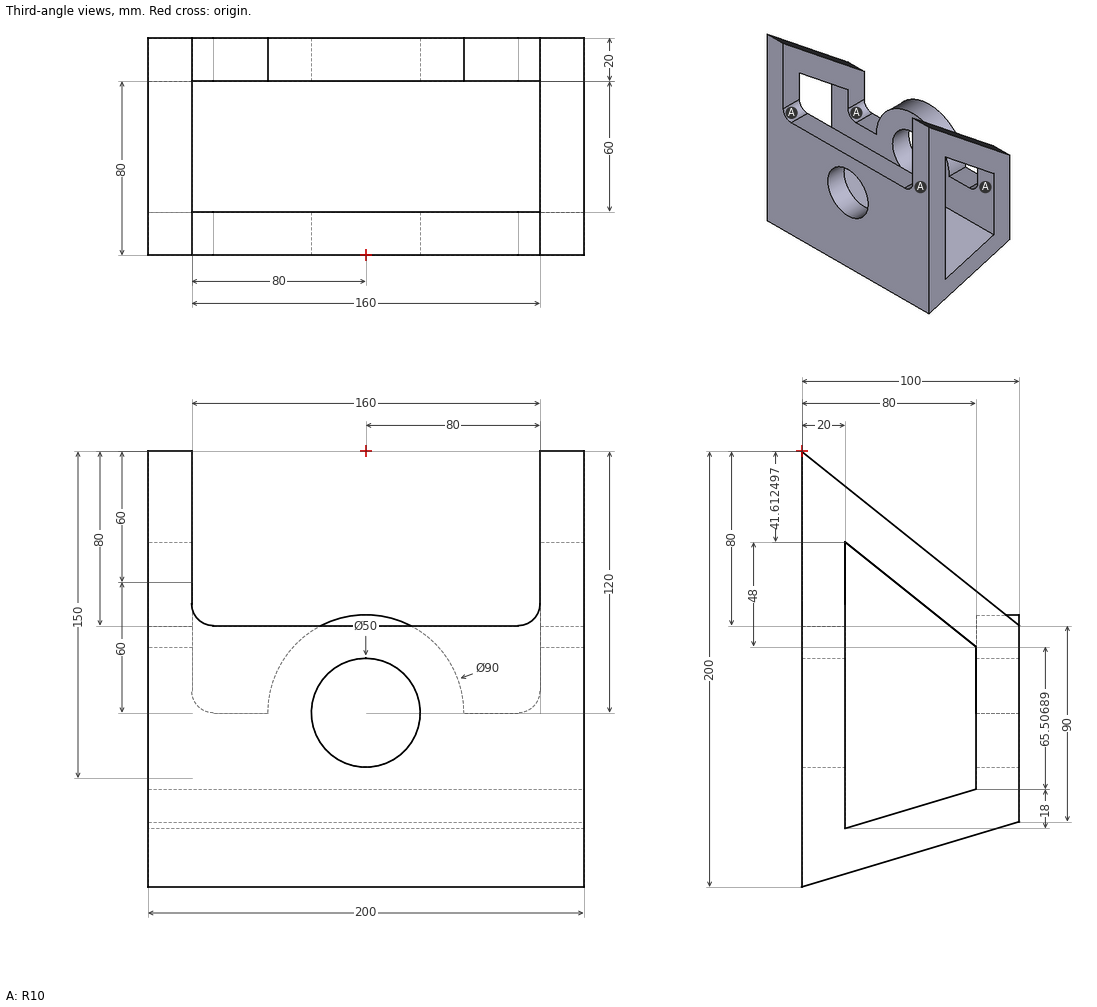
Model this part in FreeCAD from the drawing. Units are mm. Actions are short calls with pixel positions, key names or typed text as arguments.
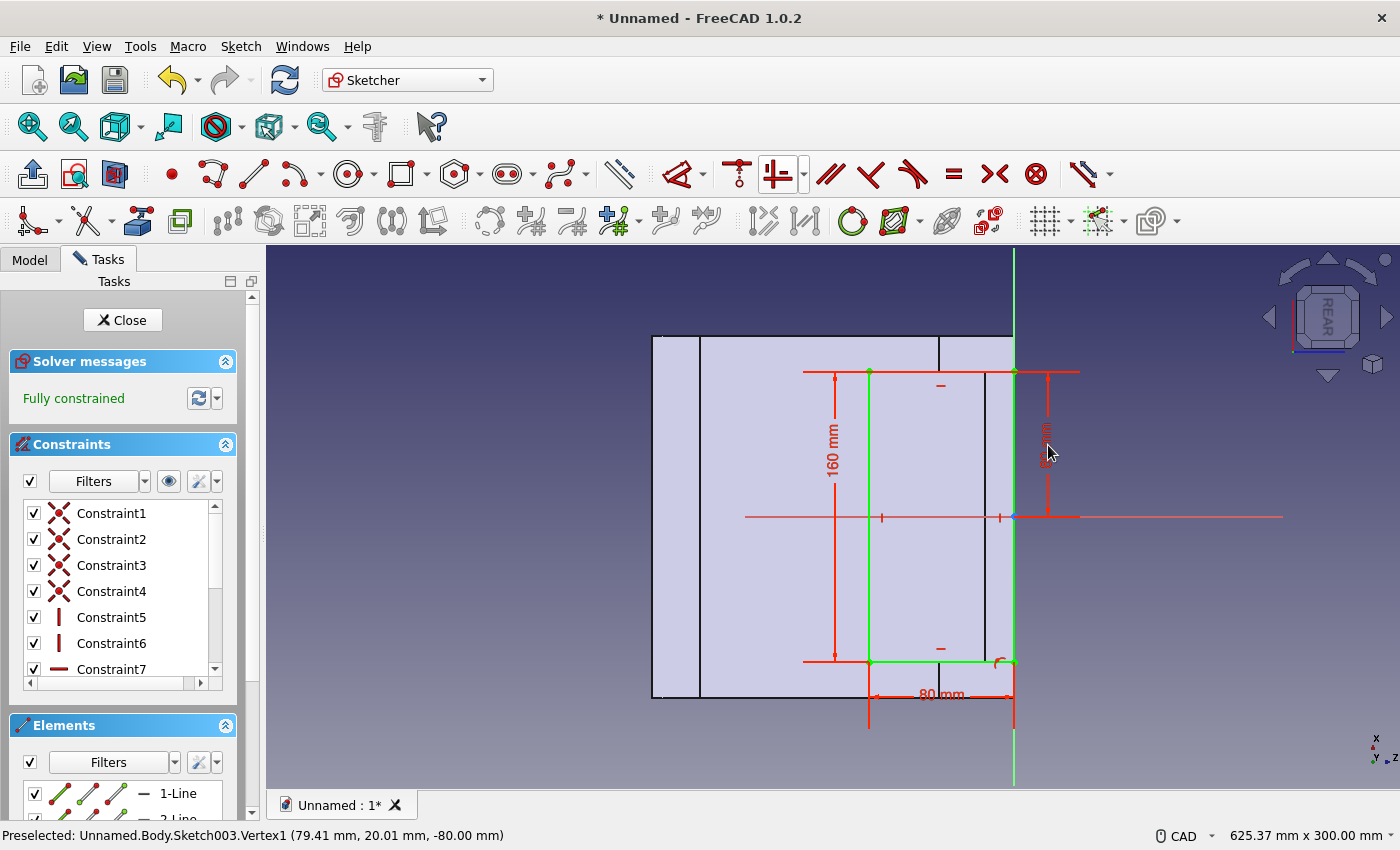
click(123, 320)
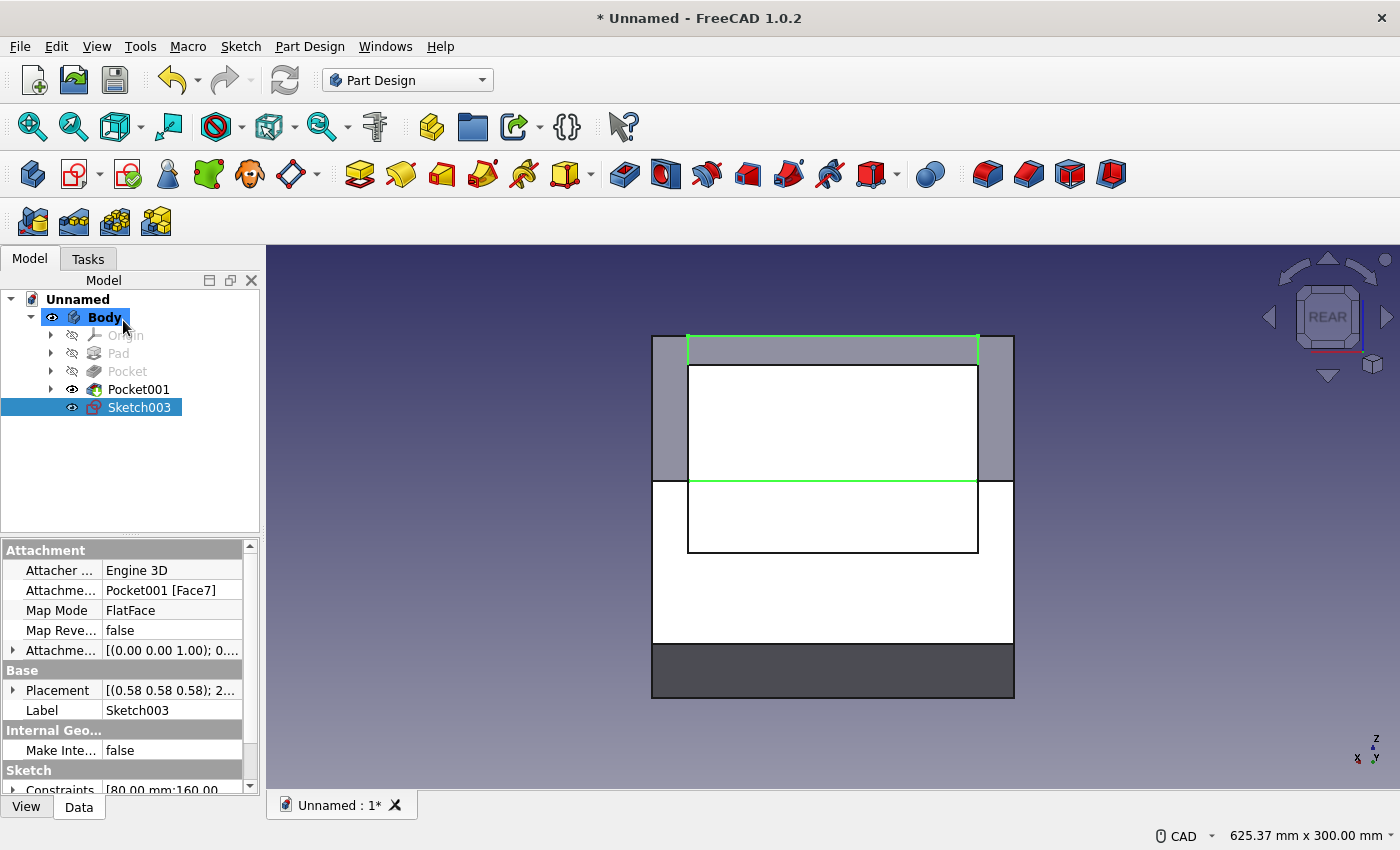
click(625, 174)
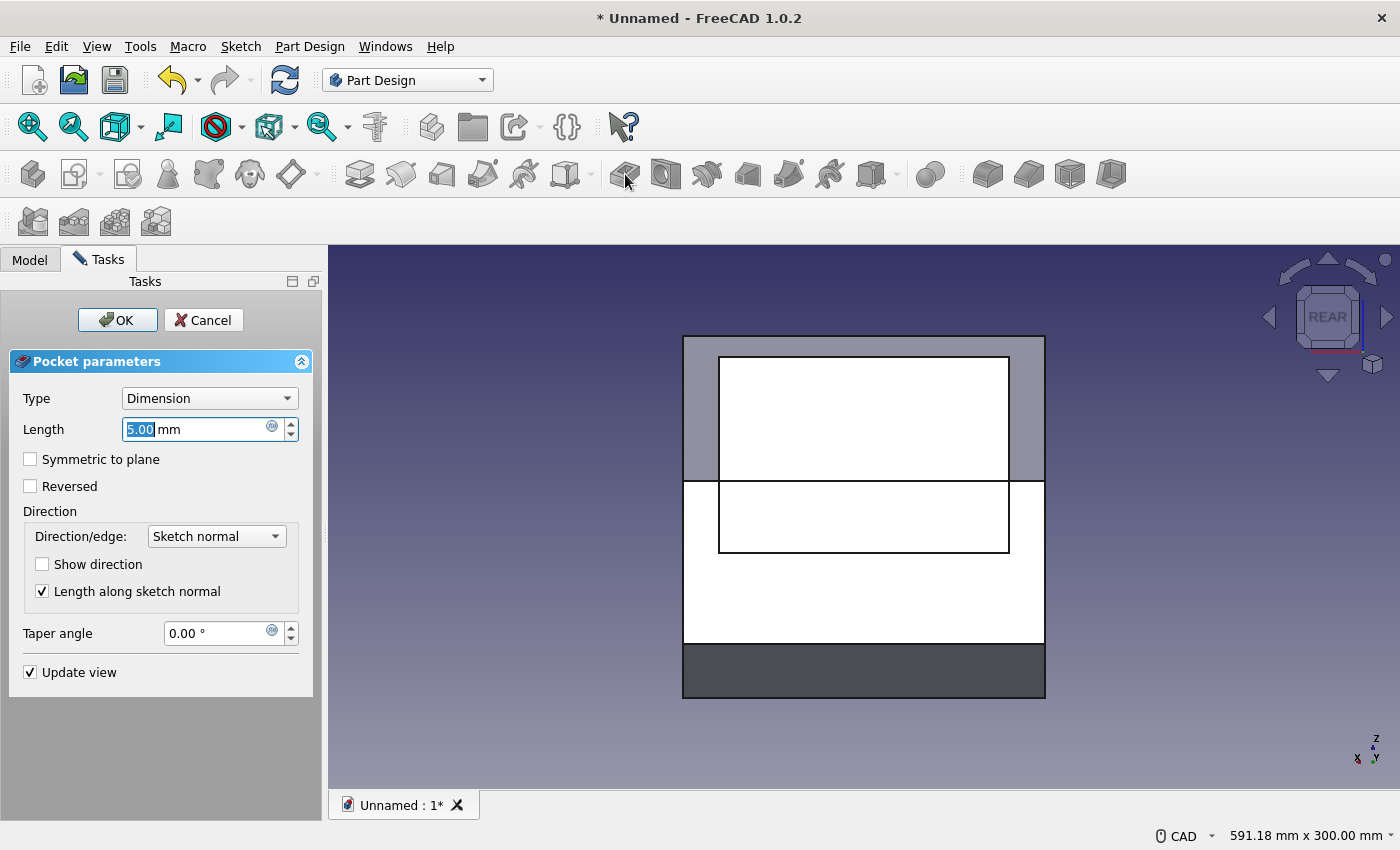
click(210, 398)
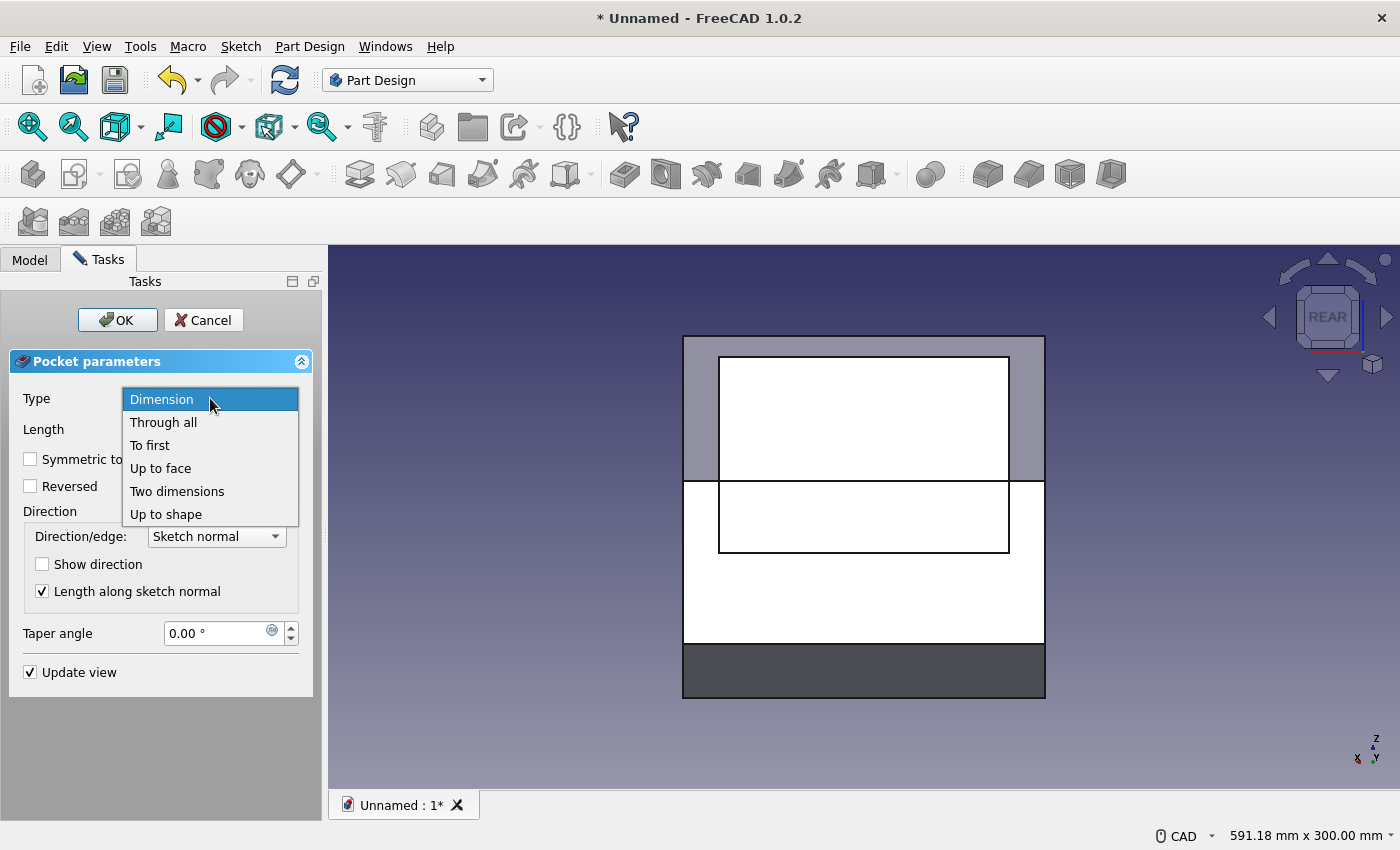
click(208, 446)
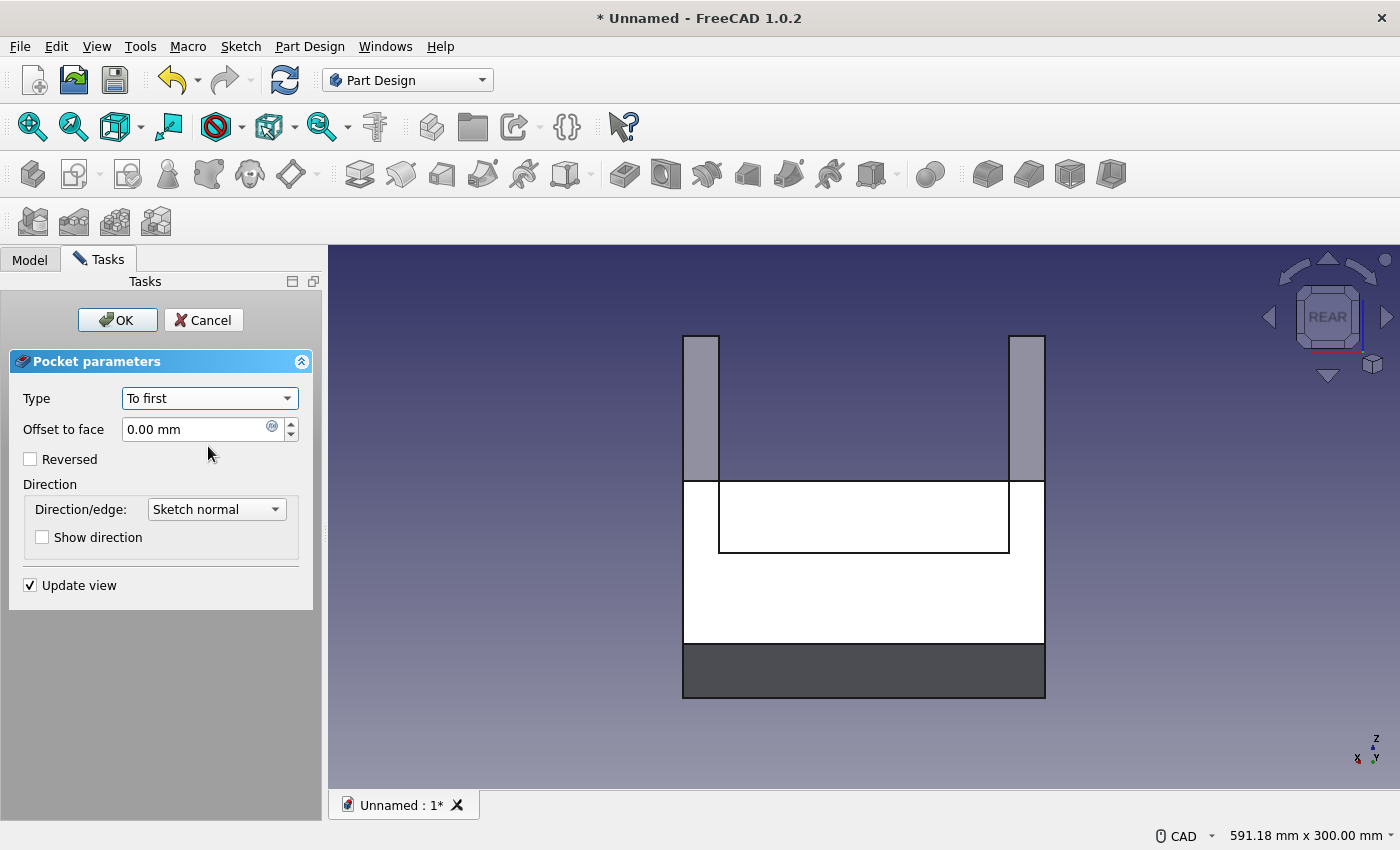
click(118, 320)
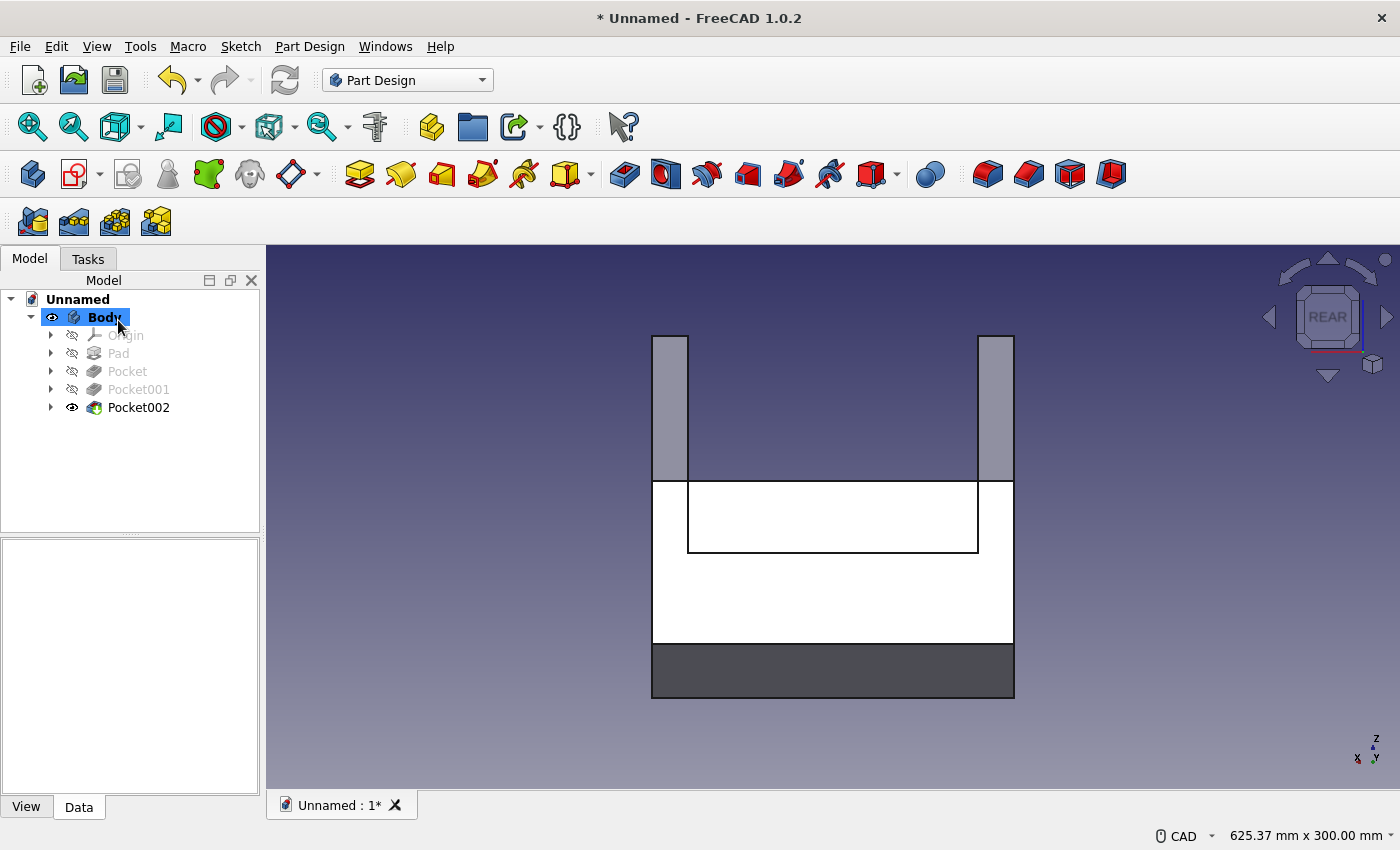
key(0)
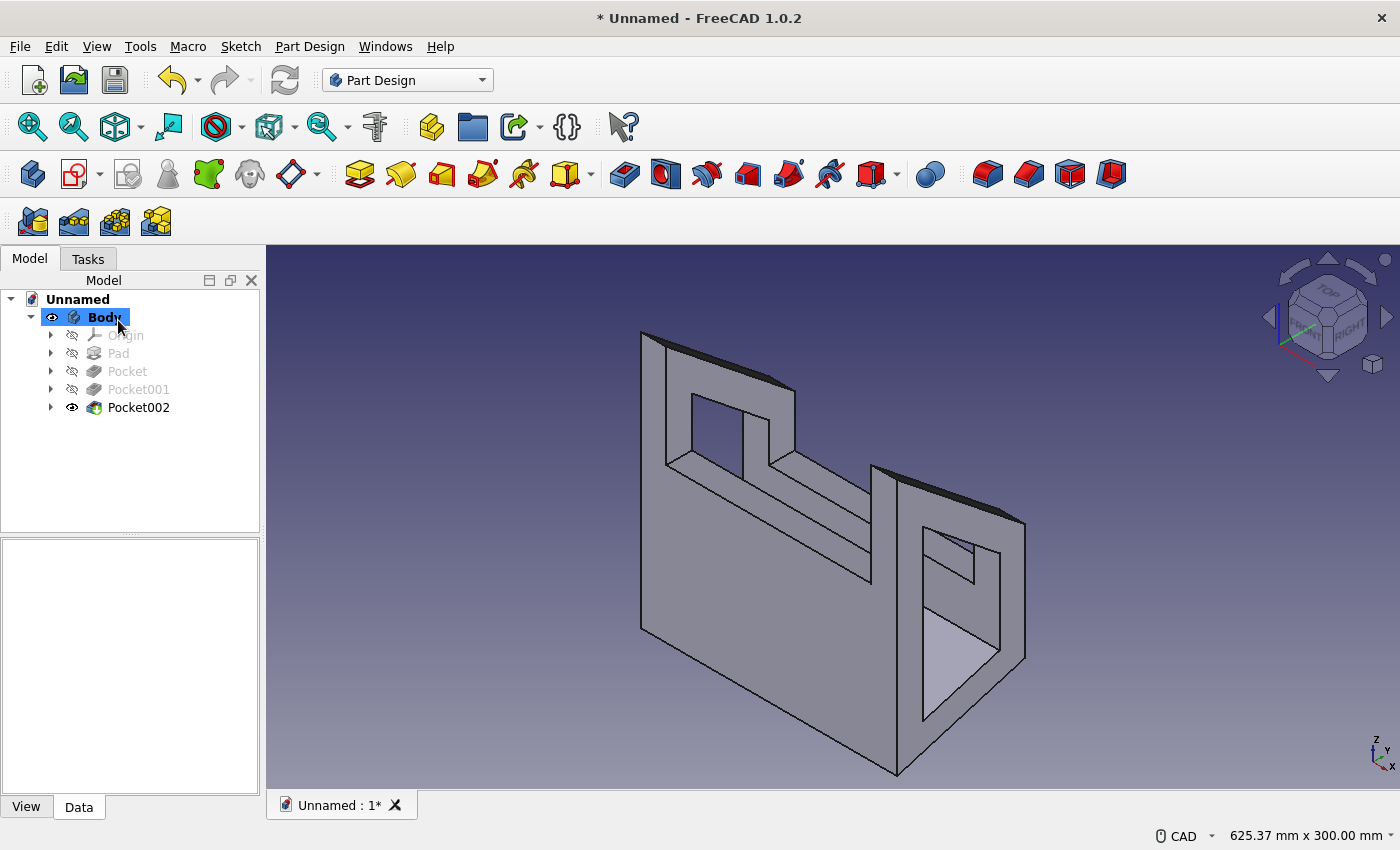
key(2)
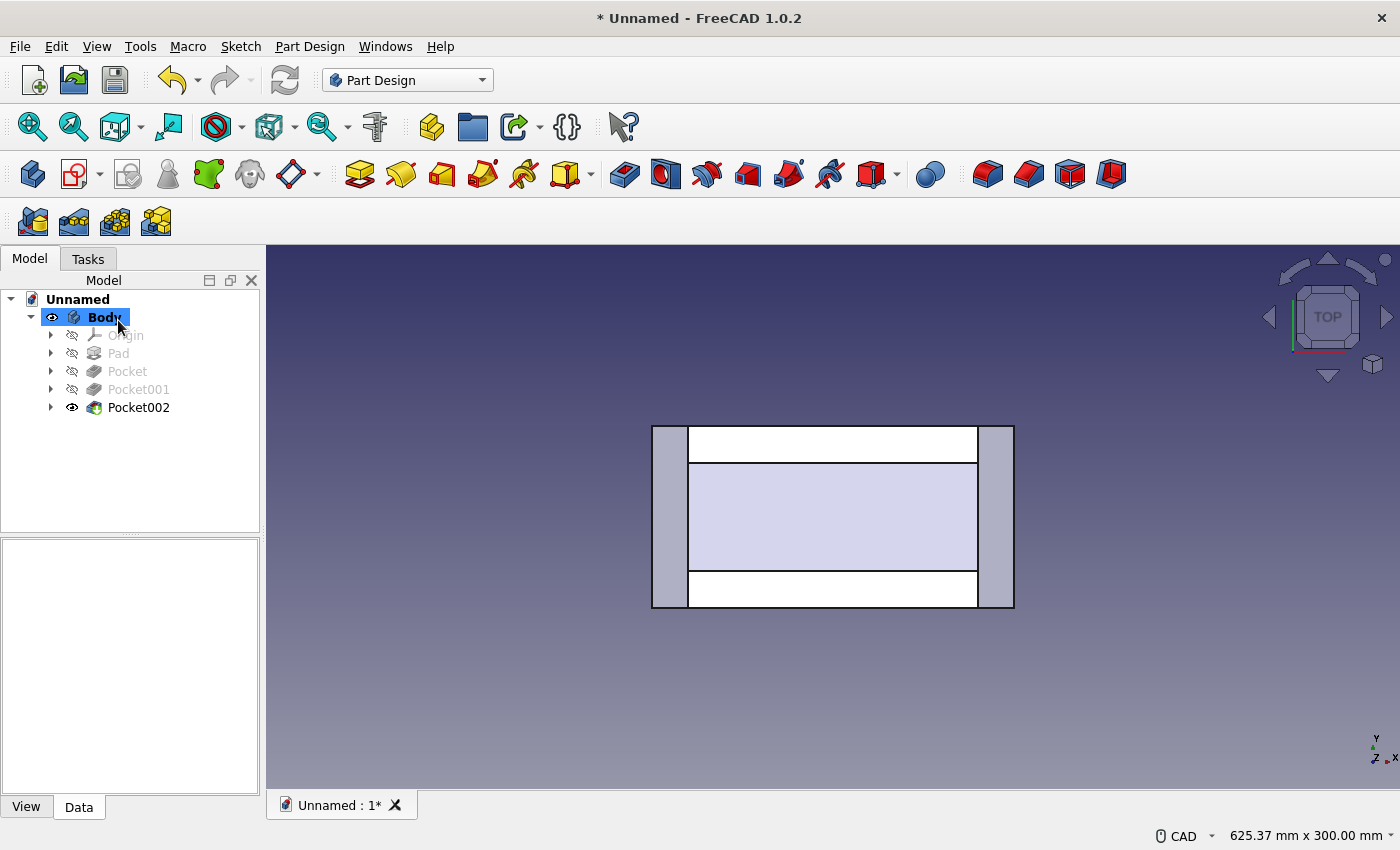
key(v)
key(f)